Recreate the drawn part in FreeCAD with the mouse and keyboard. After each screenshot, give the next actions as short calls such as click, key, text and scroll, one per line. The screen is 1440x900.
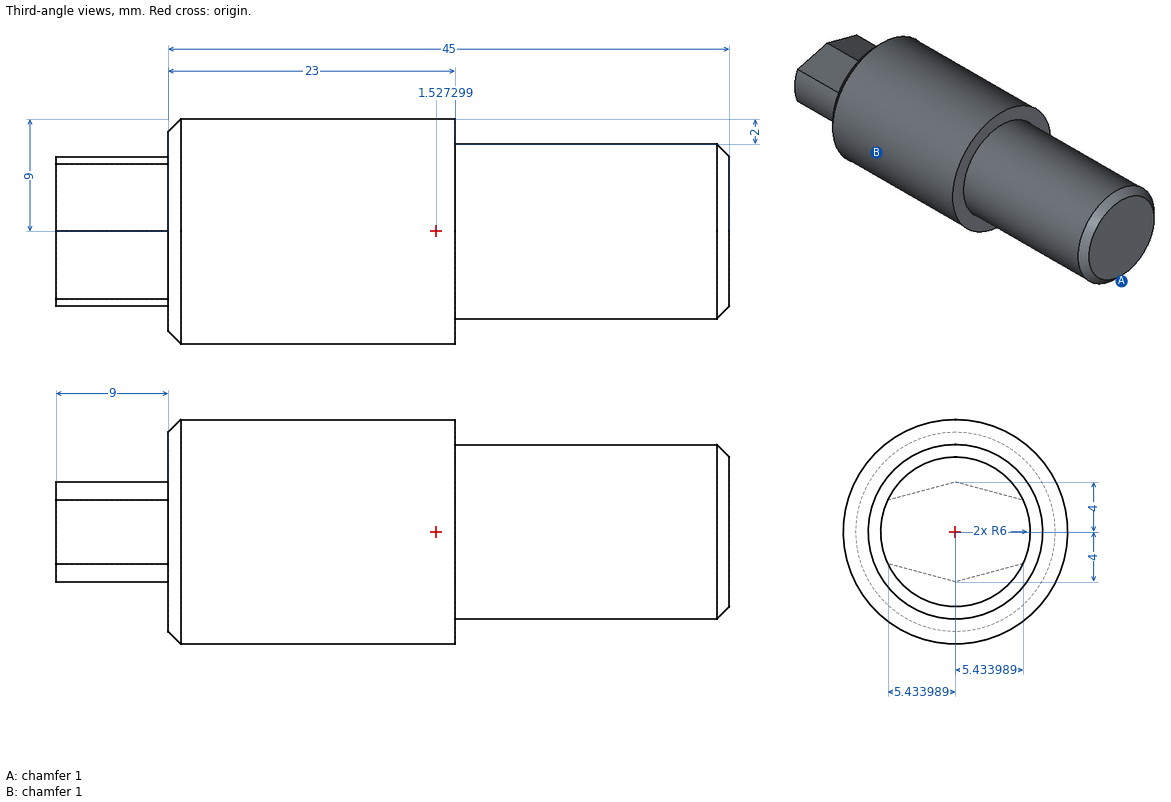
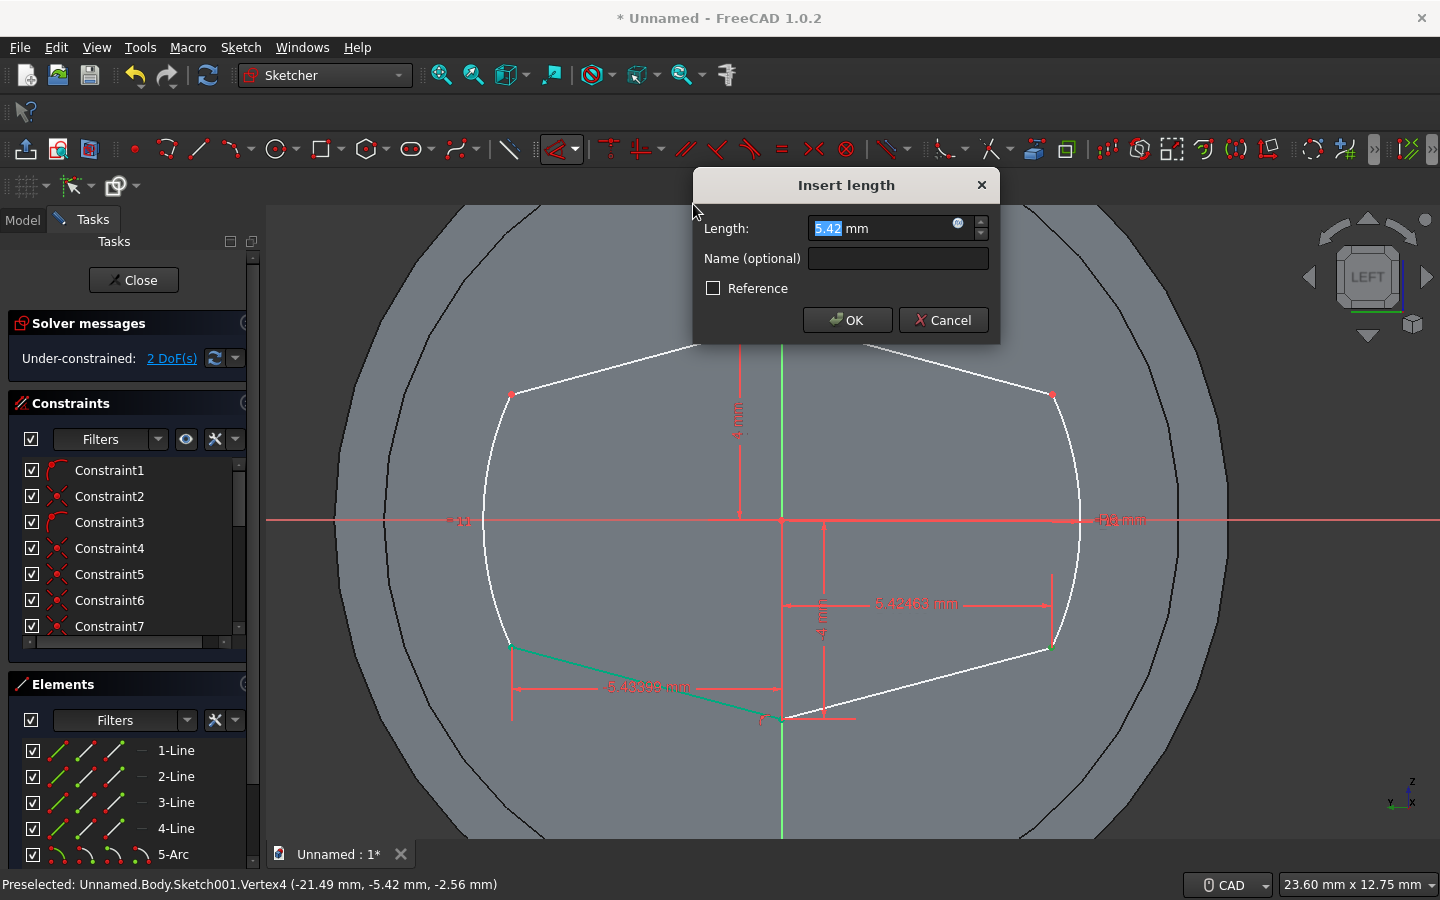
text(5.433989)
key(Return)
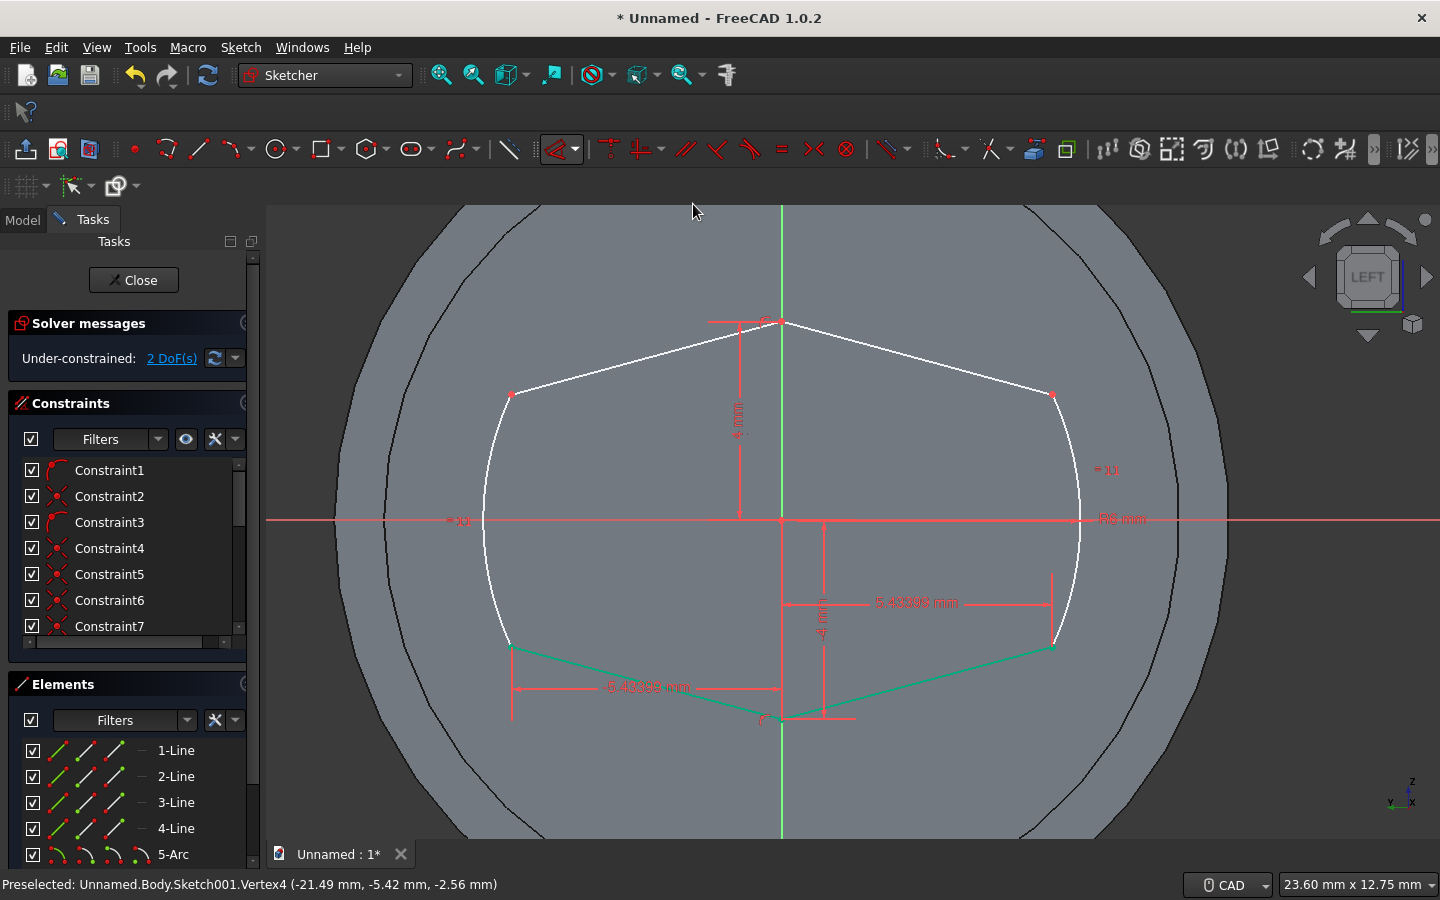
click(1053, 395)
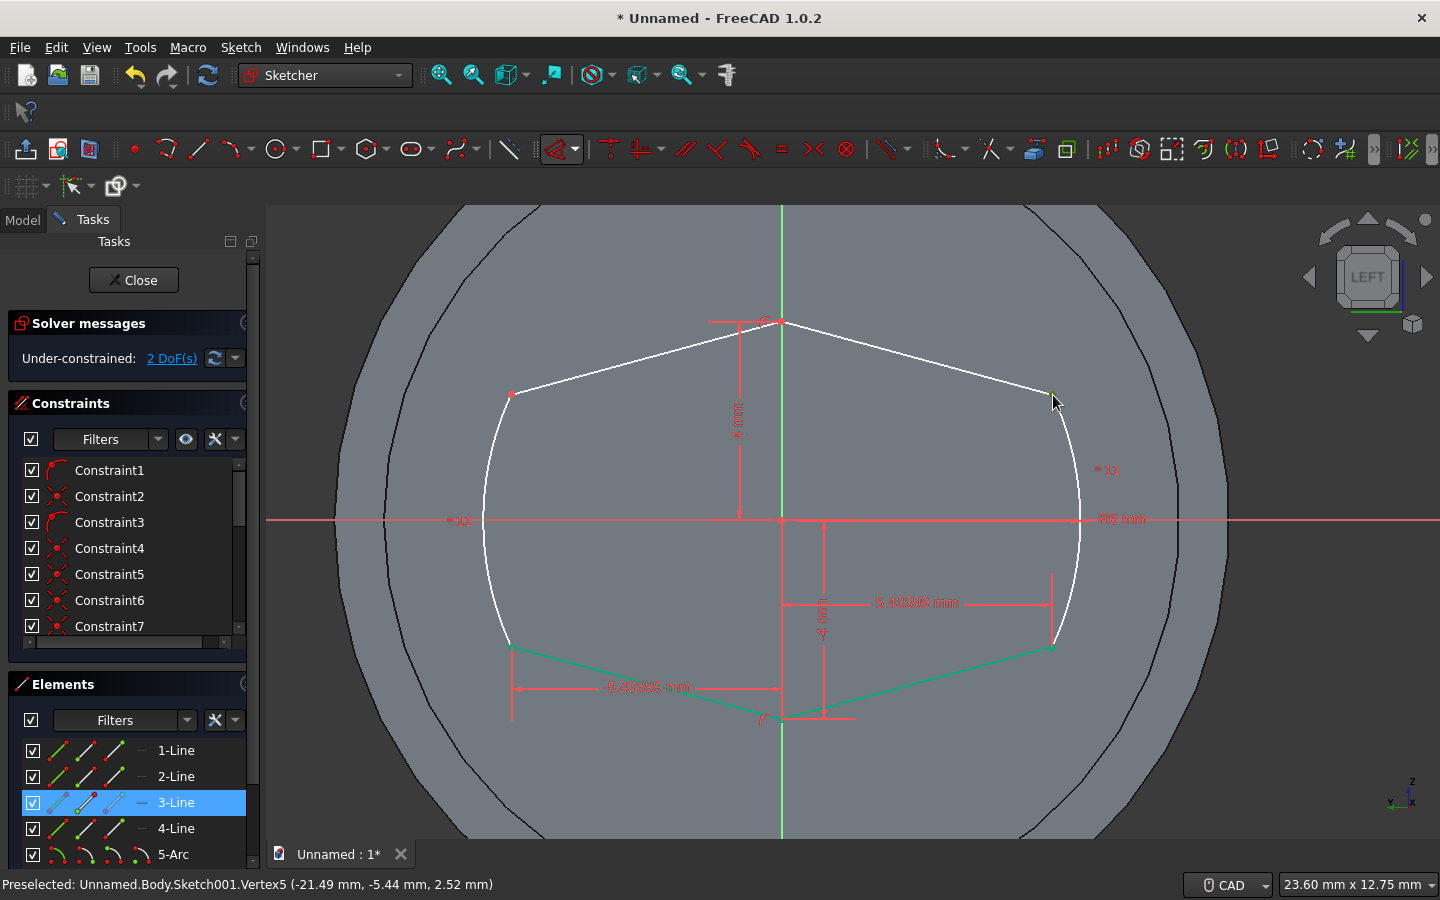
click(578, 150)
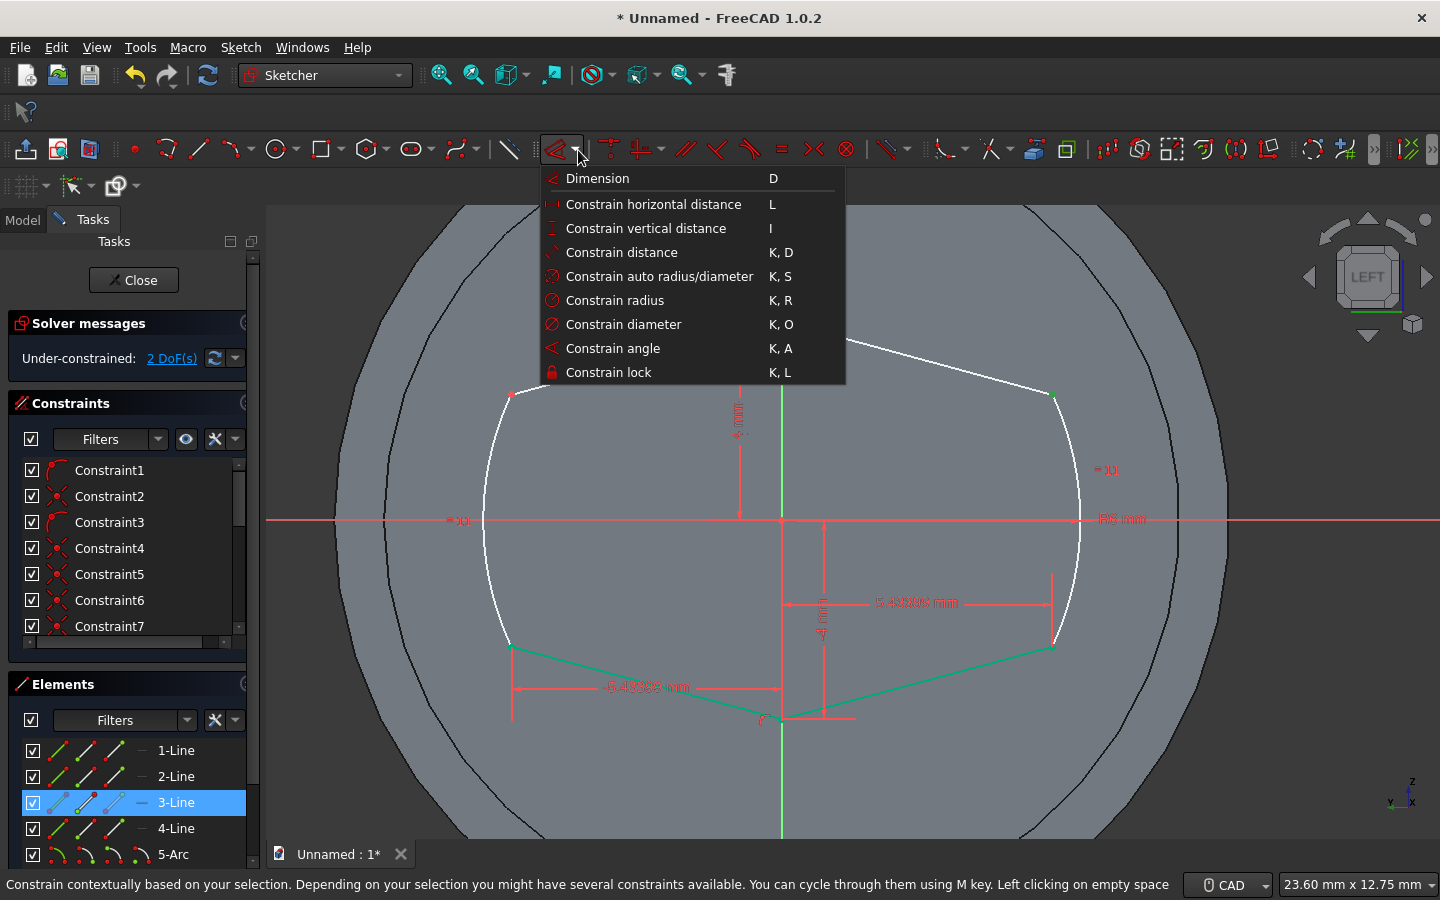
click(693, 204)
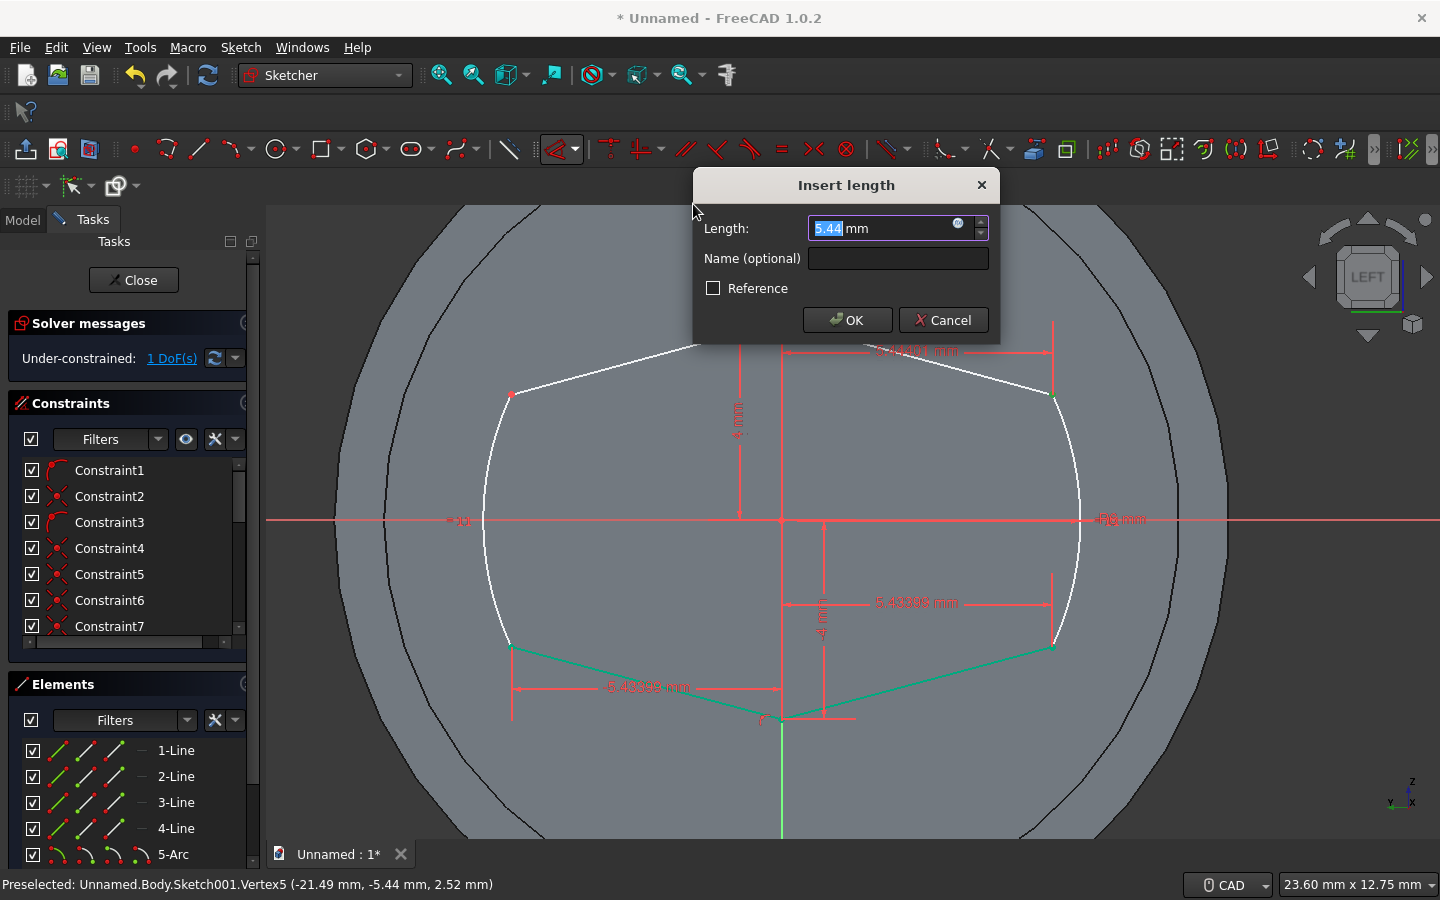
text(5.433989)
key(Return)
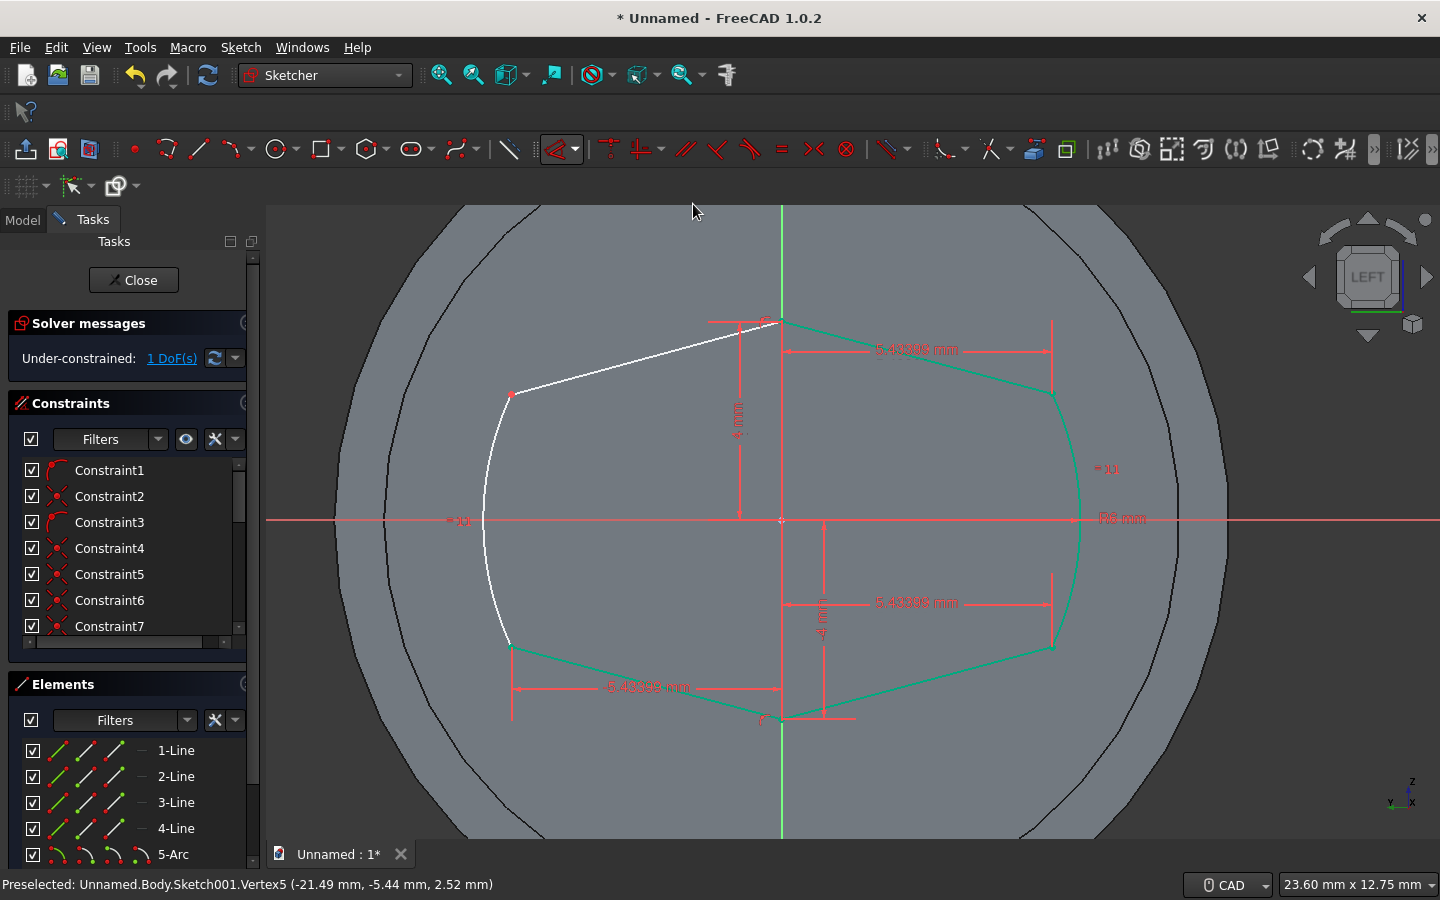
click(511, 395)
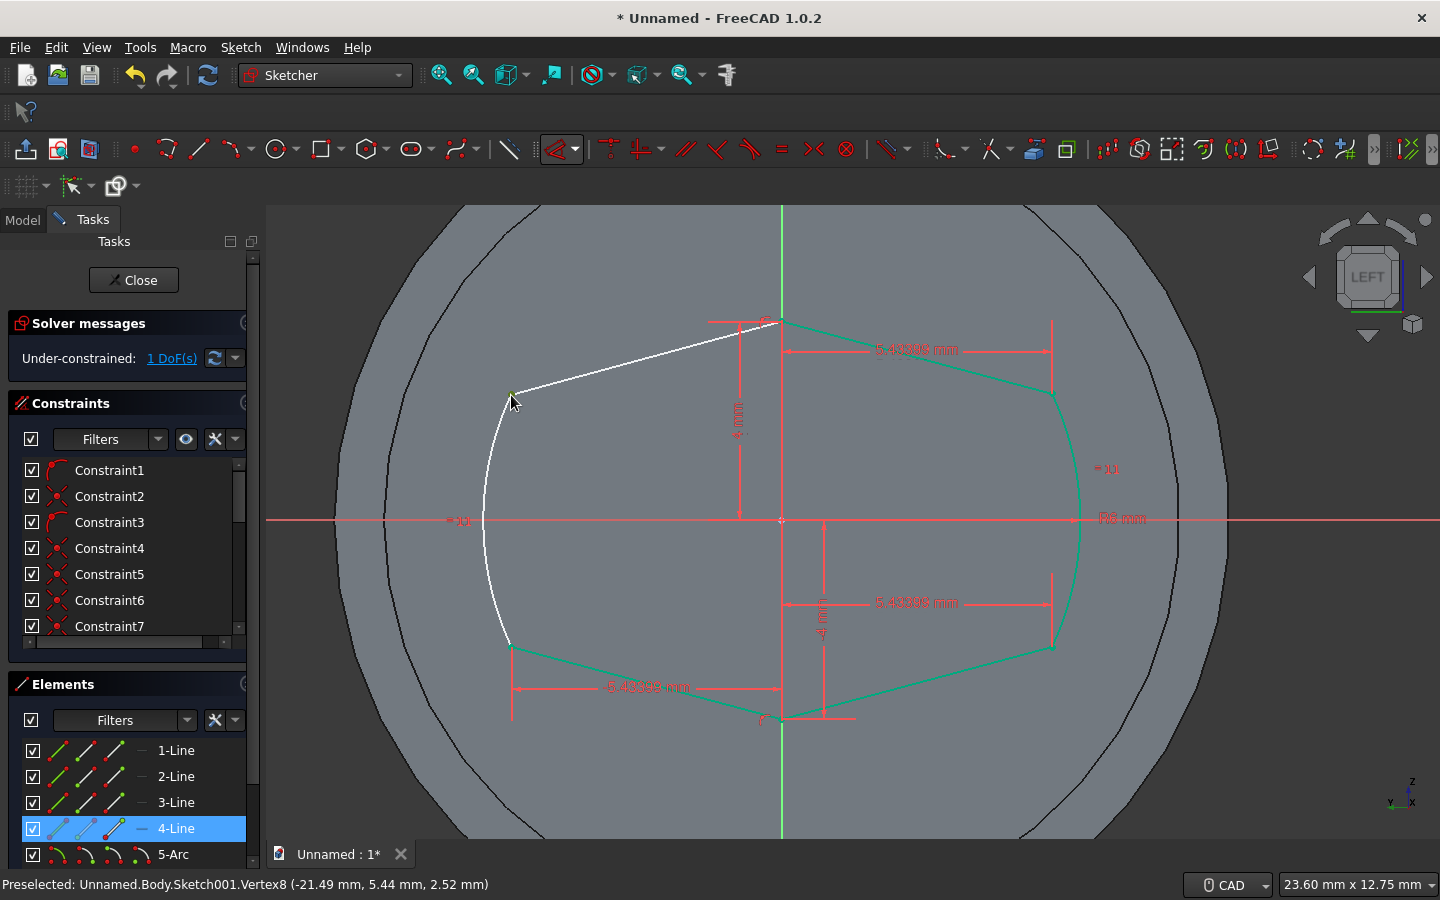
key(l)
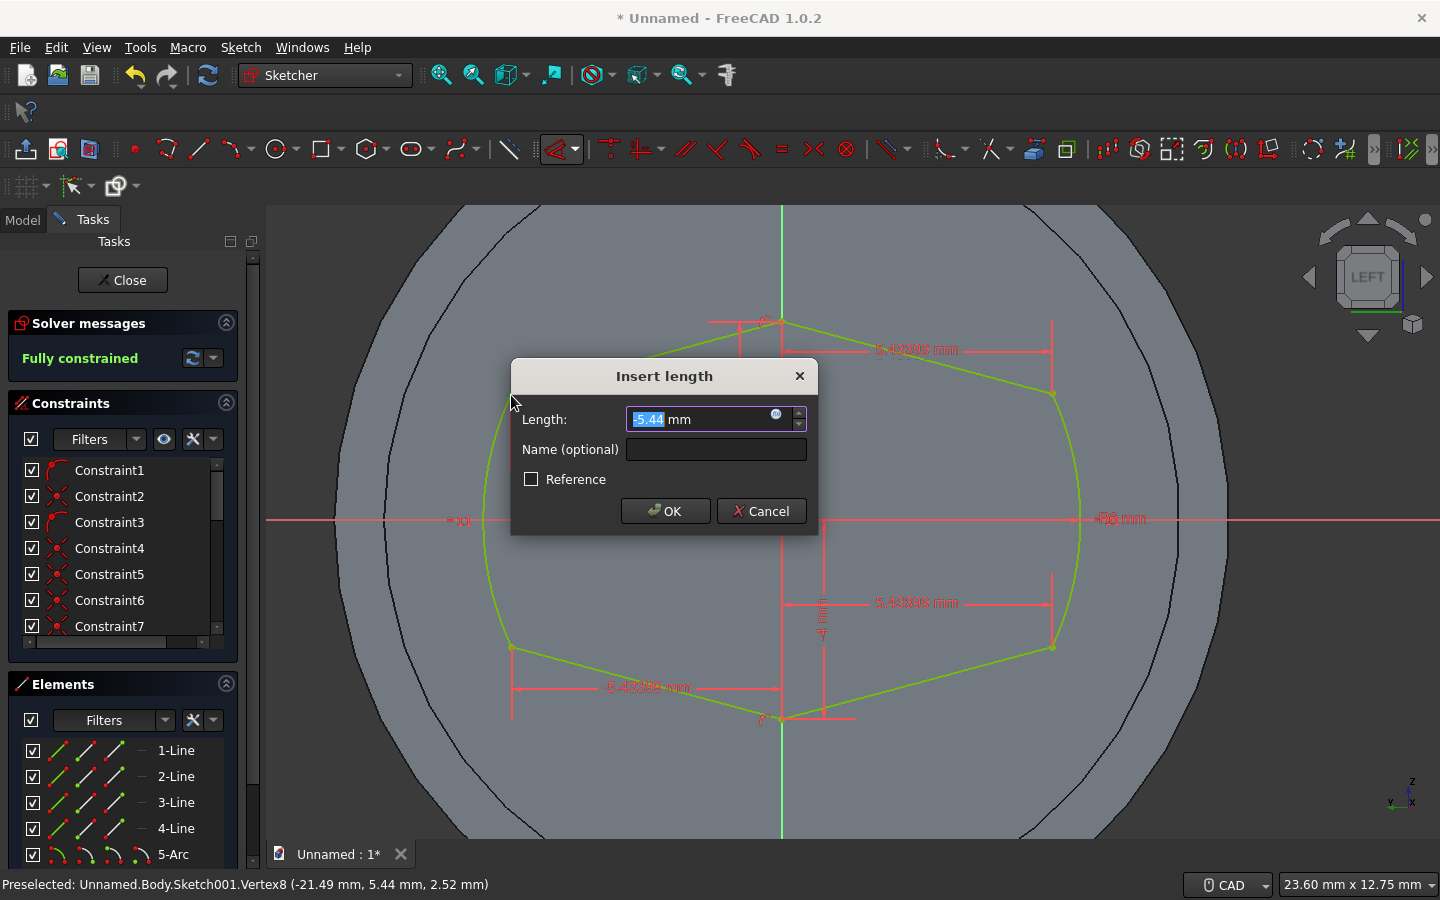
text(-5.433989)
key(Return)